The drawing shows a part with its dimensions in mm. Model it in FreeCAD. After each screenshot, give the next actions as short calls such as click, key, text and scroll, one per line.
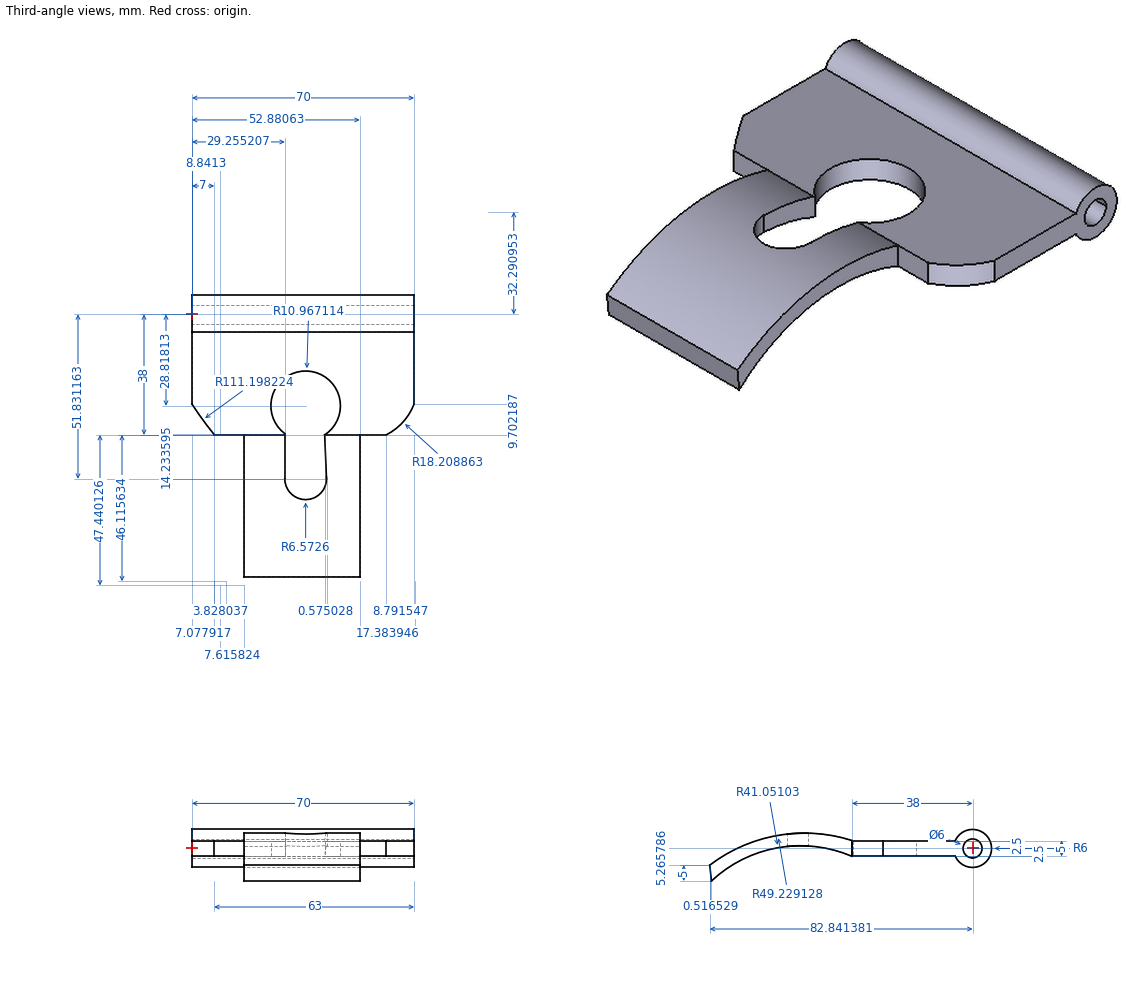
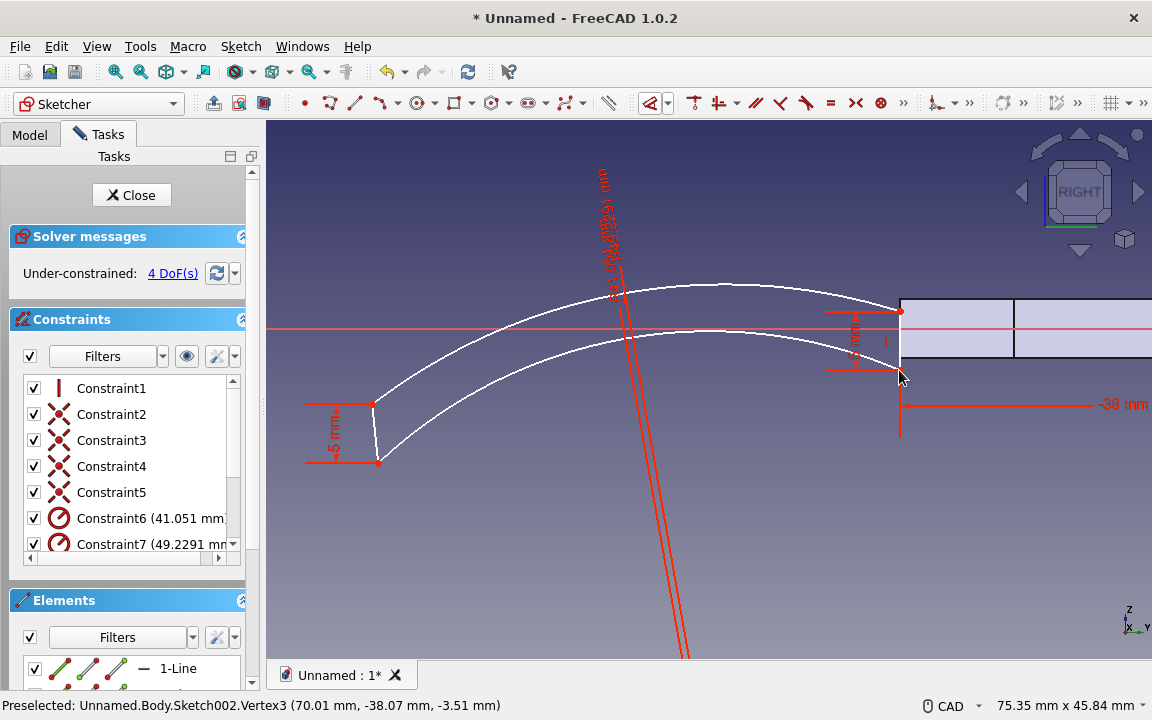
scroll(900, 370, up, 2)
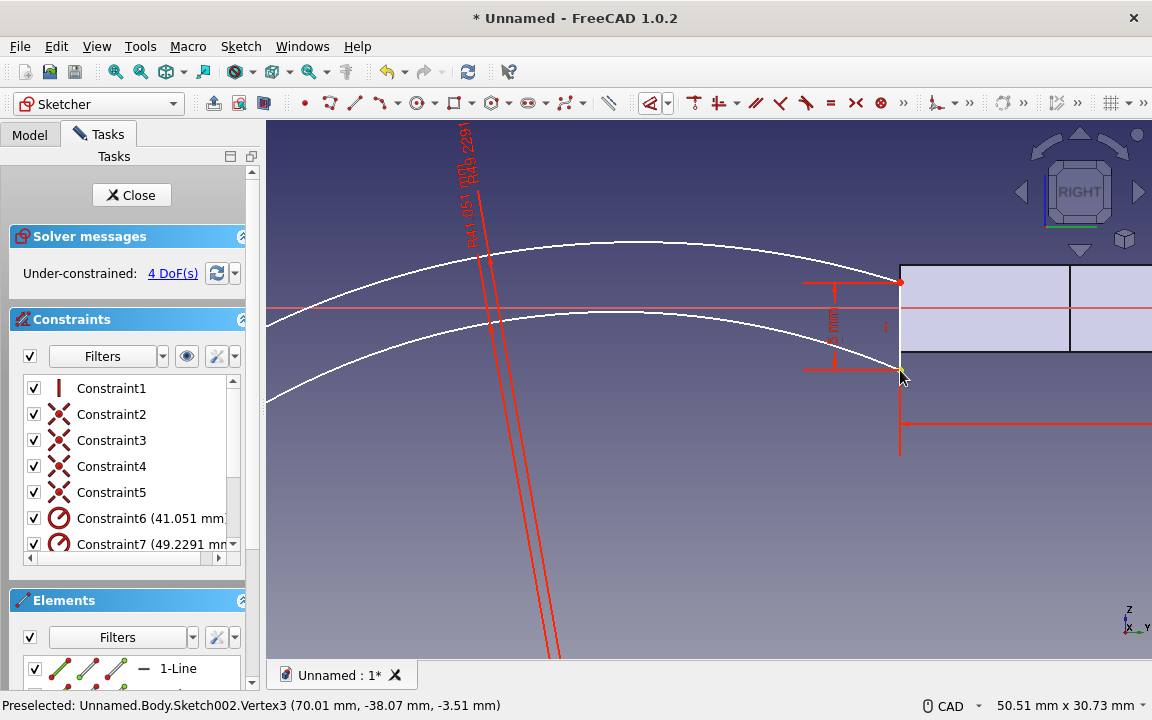
click(900, 370)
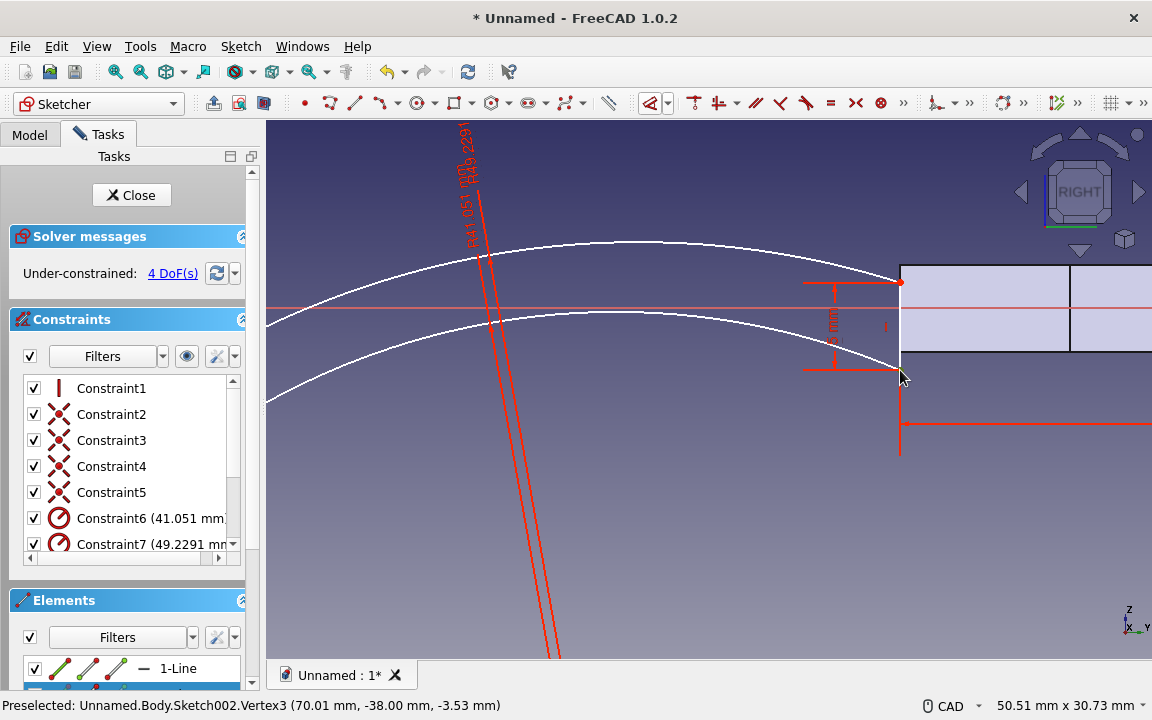
key(i)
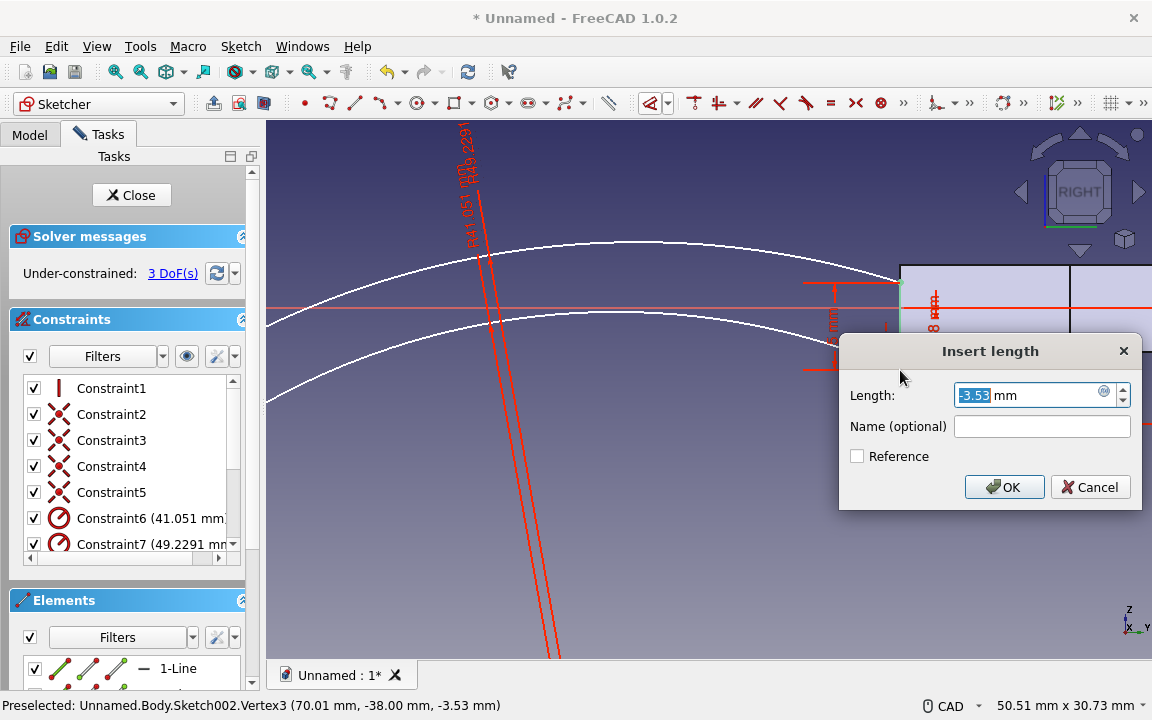
text(-2.5)
key(Return)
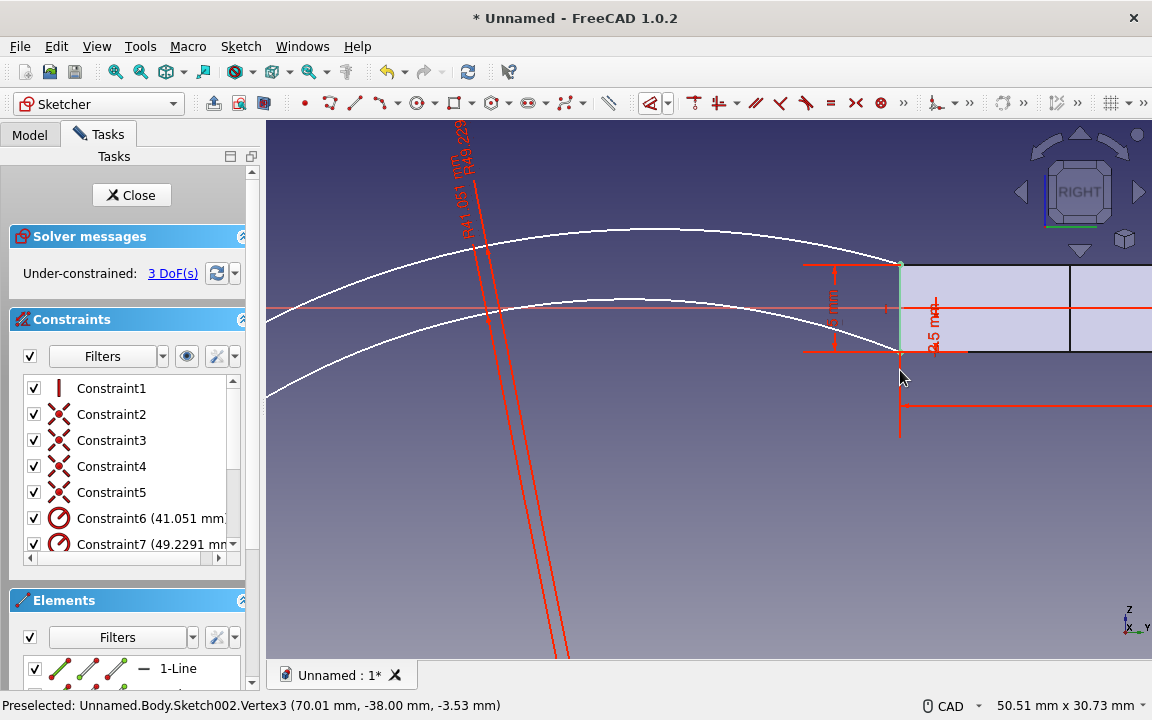
scroll(524, 405, down, 5)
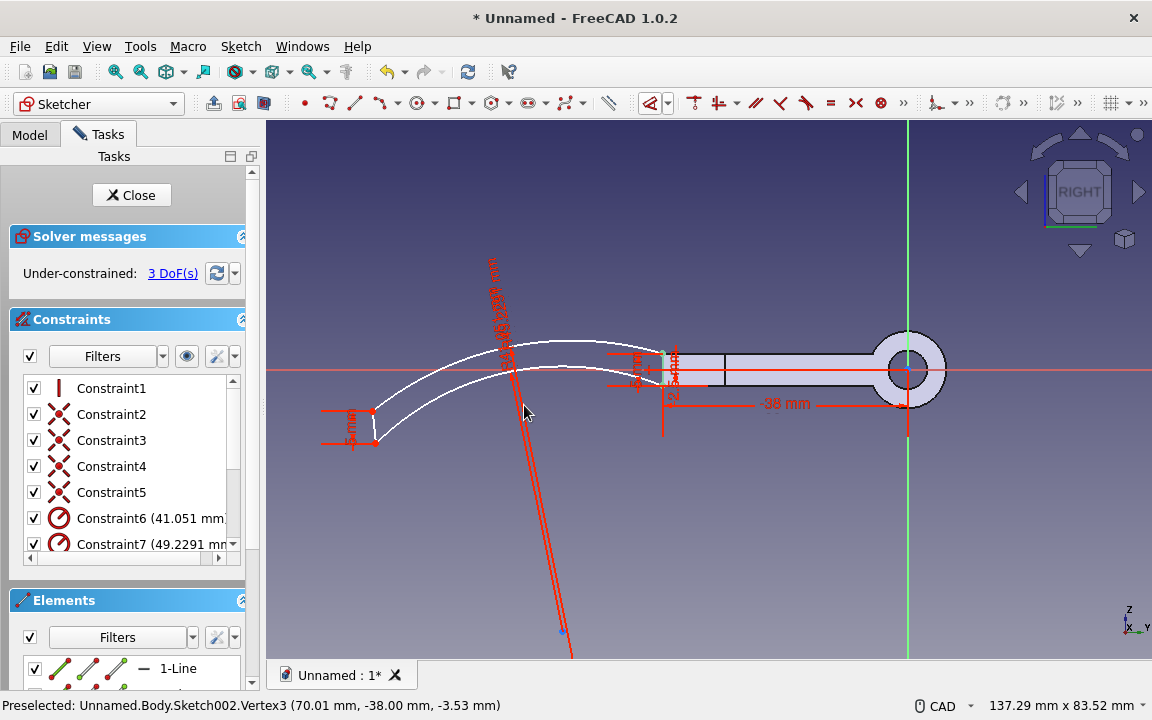
click(373, 411)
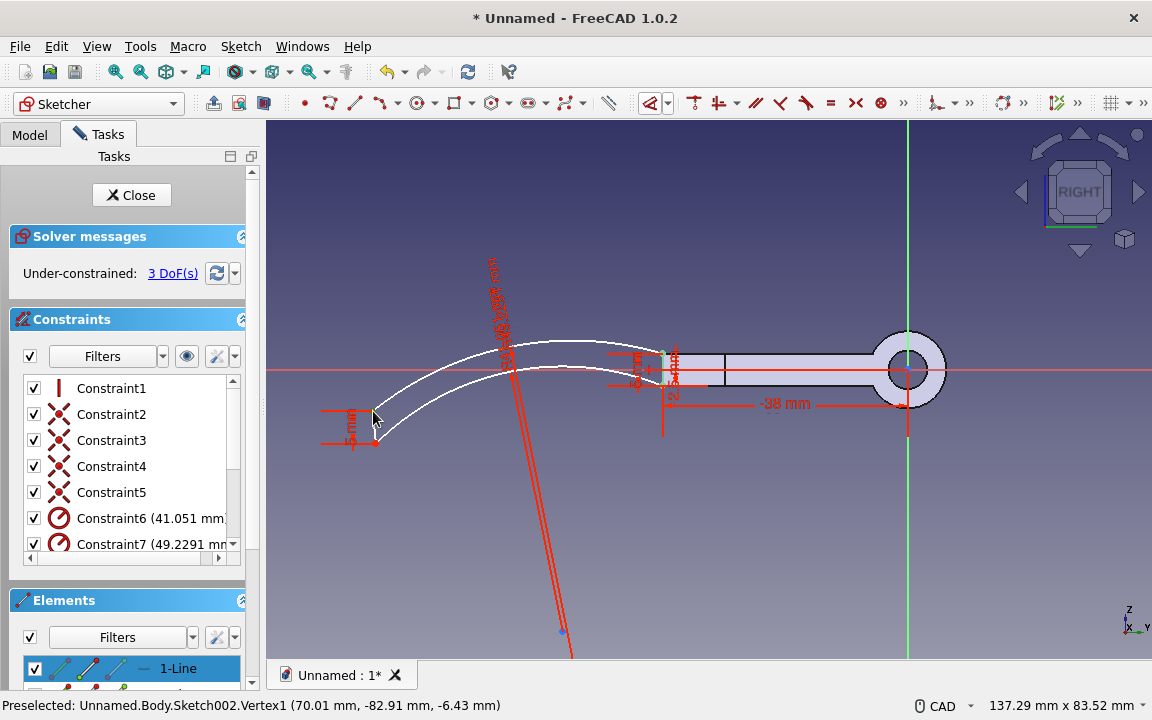
key(i)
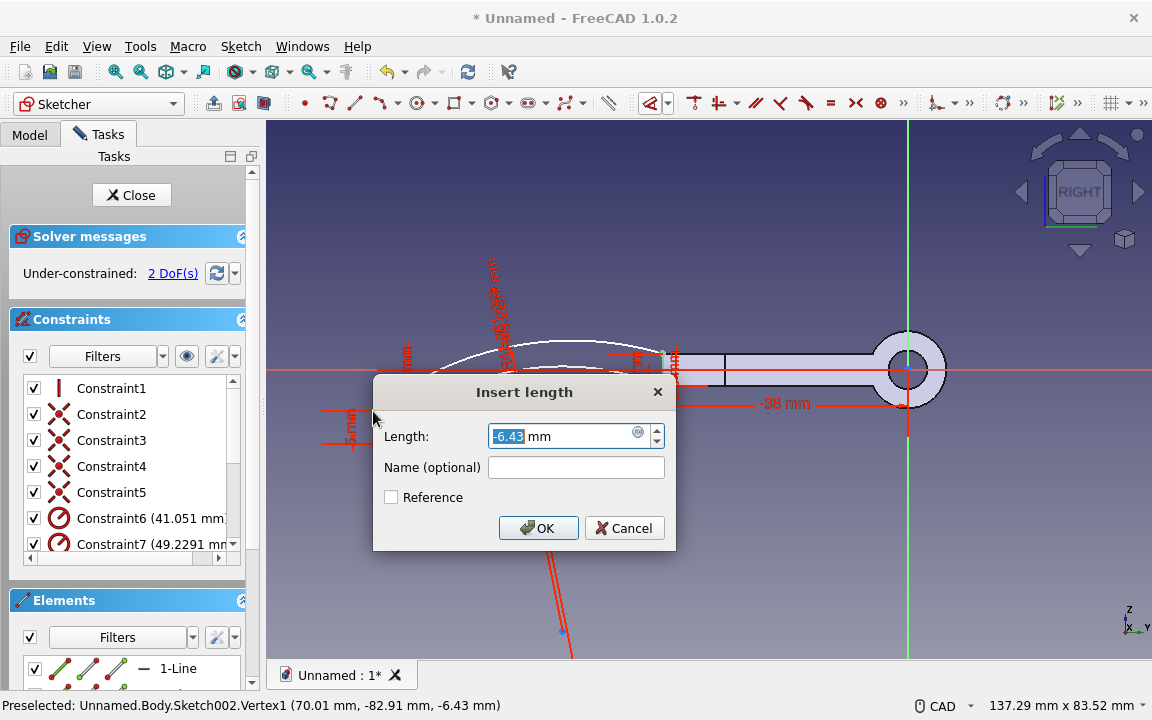
text(-5.265786)
key(Return)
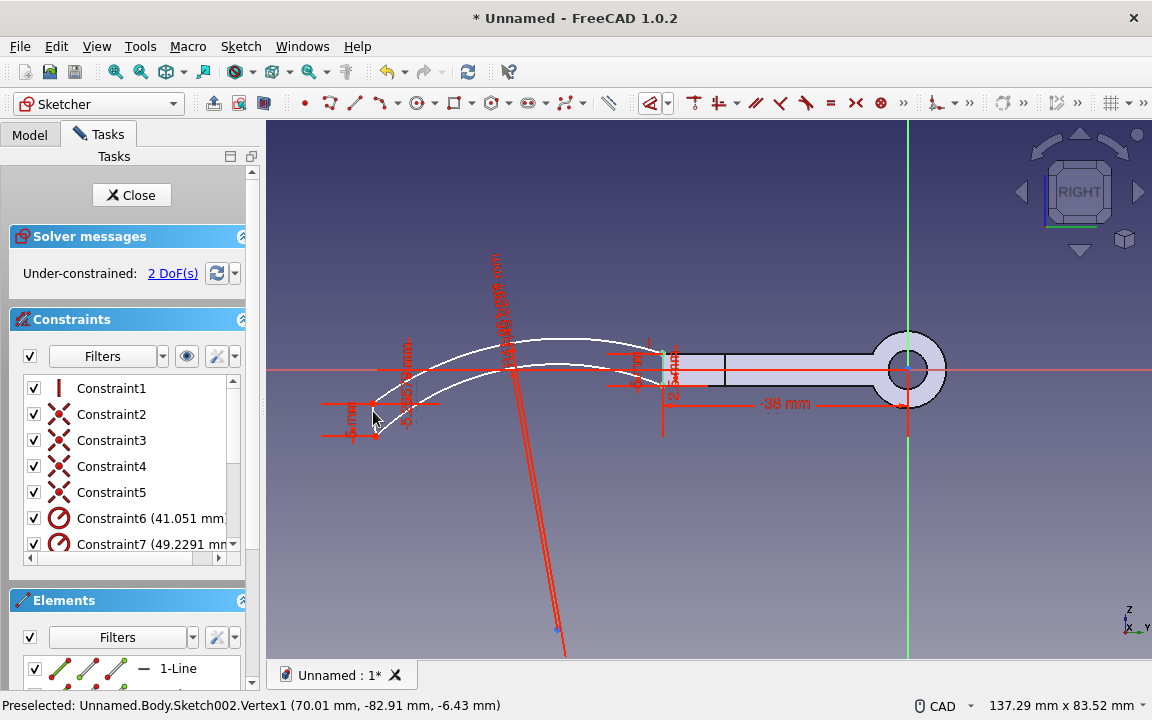
scroll(374, 413, up, 13)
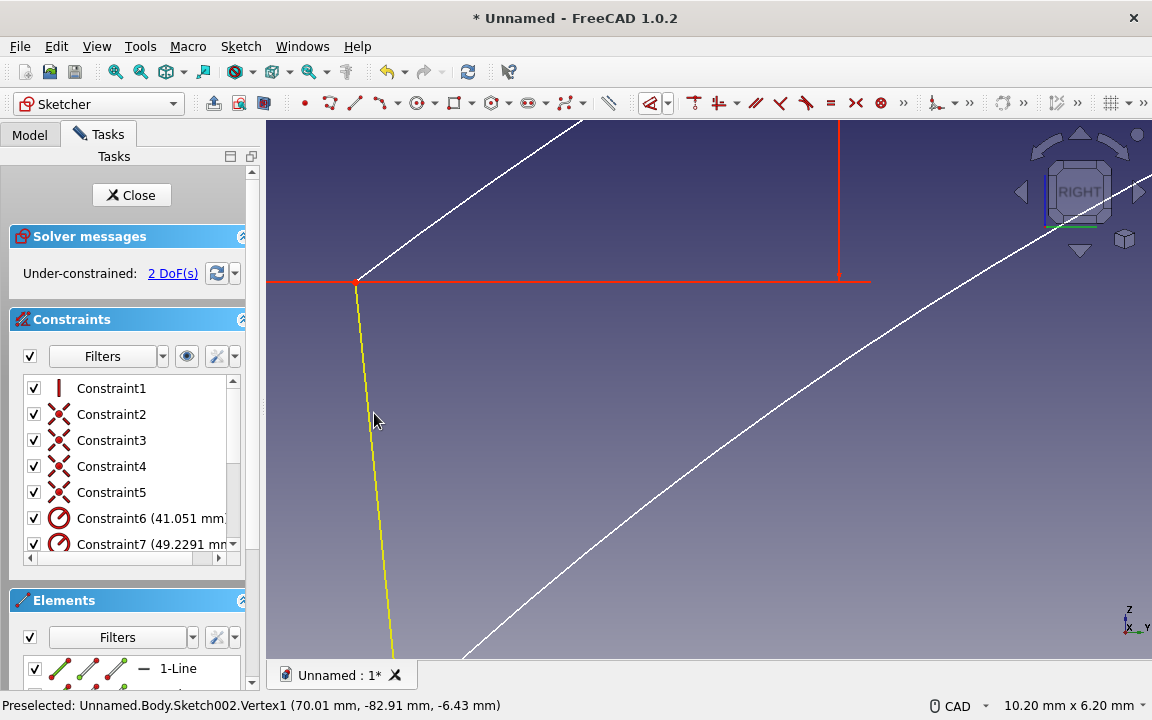
click(369, 412)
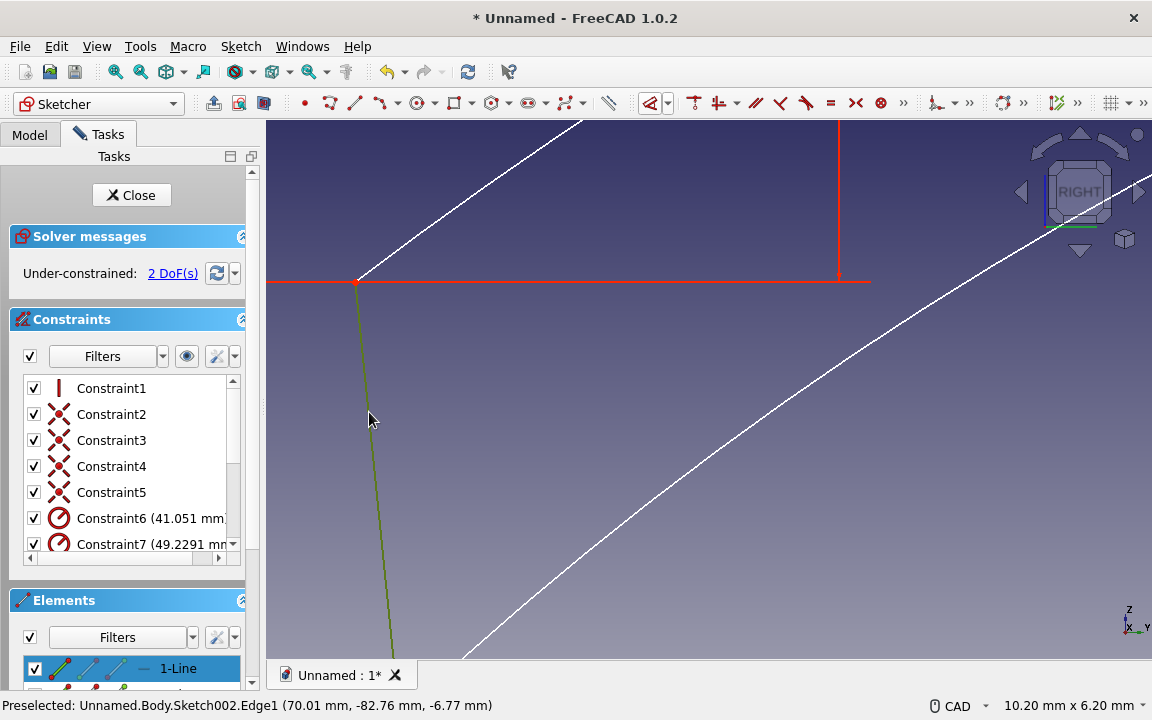
click(668, 104)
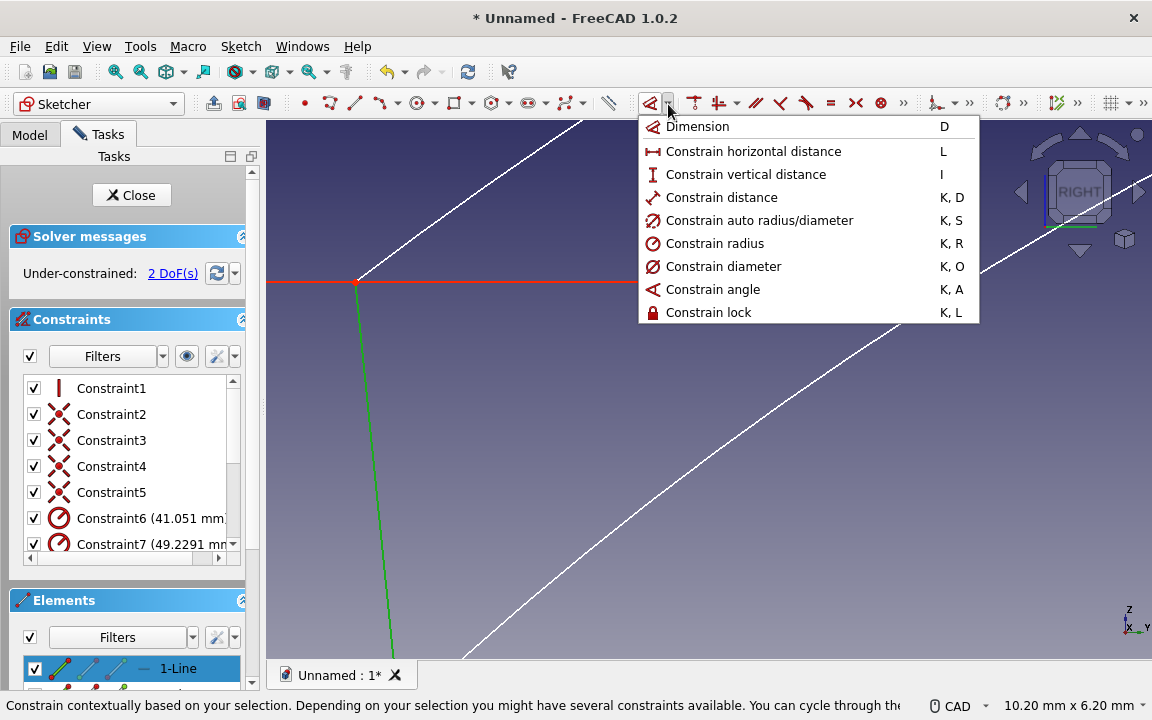
click(809, 152)